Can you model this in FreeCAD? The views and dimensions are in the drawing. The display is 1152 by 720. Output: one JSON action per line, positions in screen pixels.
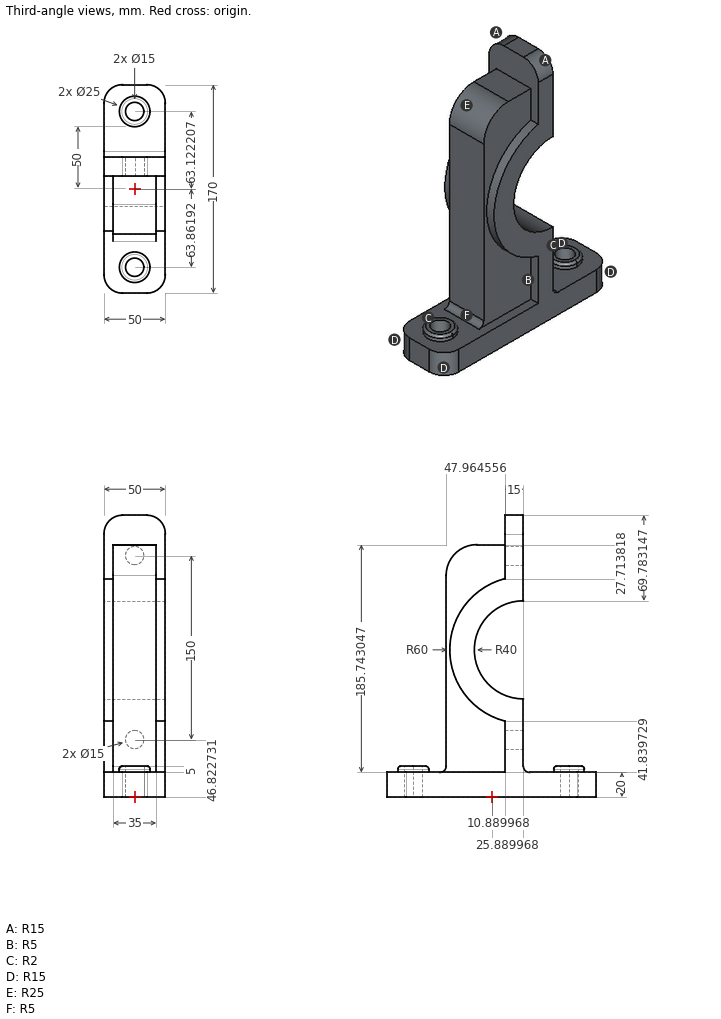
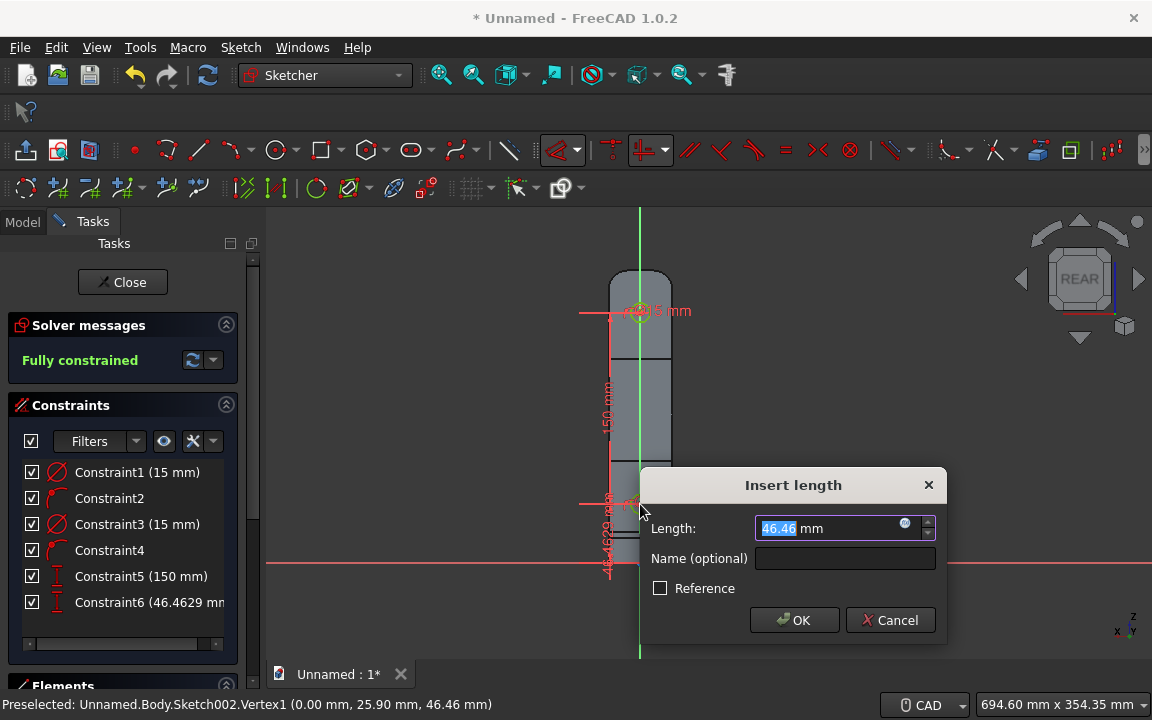
{"action": "type", "text": "46.822731"}
{"action": "key", "text": "Return"}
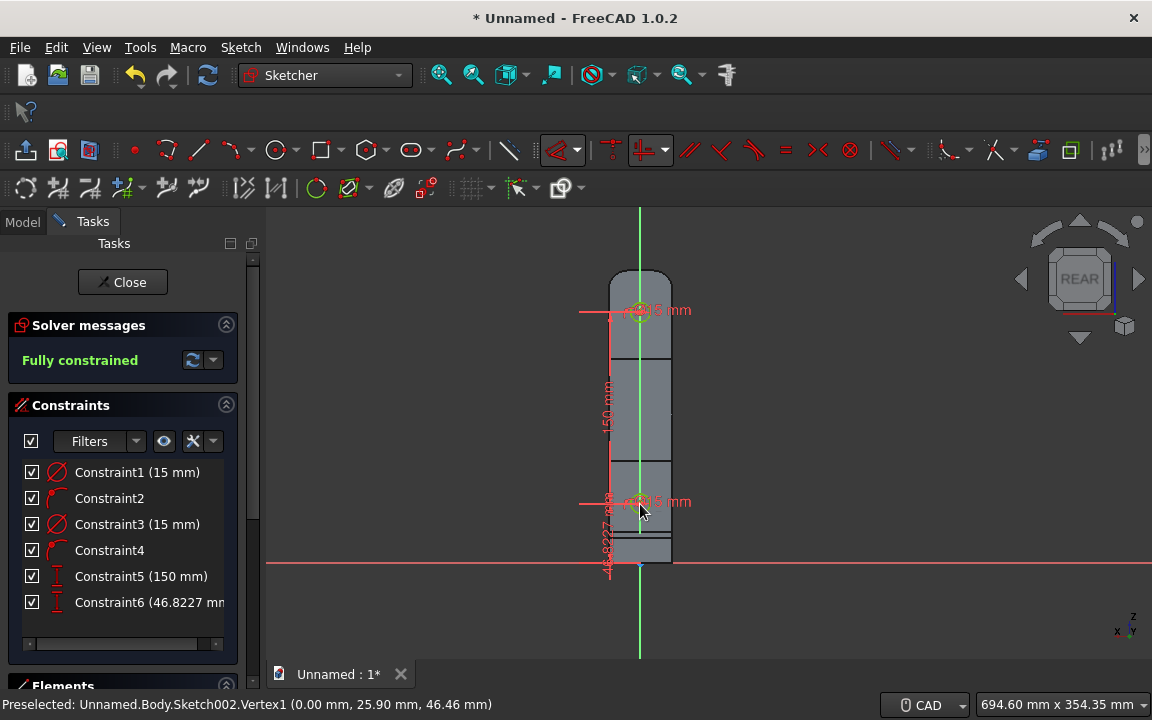
{"action": "left_click", "coordinate": [123, 282]}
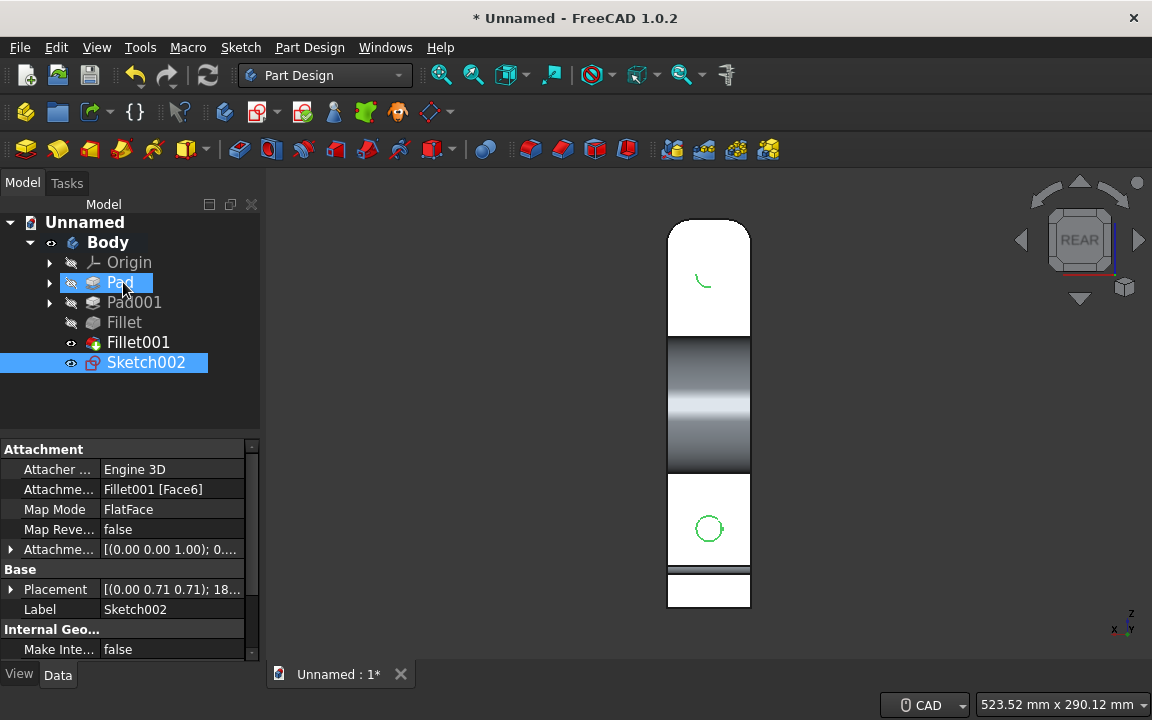
{"action": "left_click", "coordinate": [240, 150]}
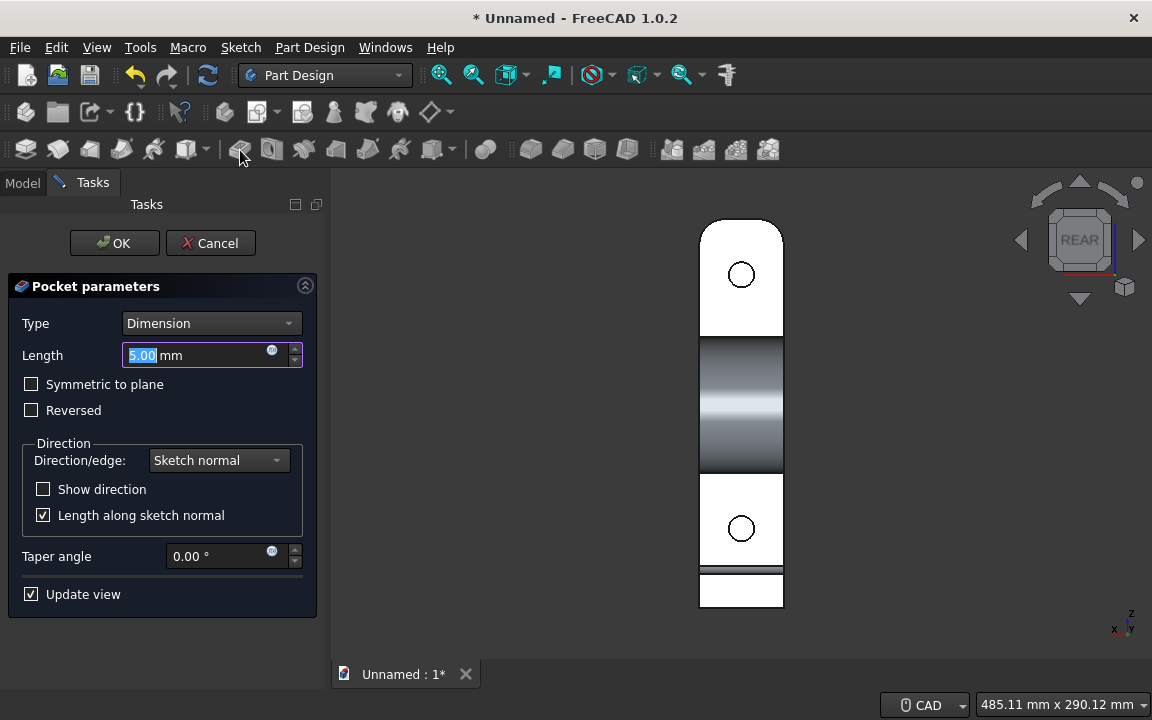
{"action": "type", "text": "50"}
{"action": "key", "text": "Tab"}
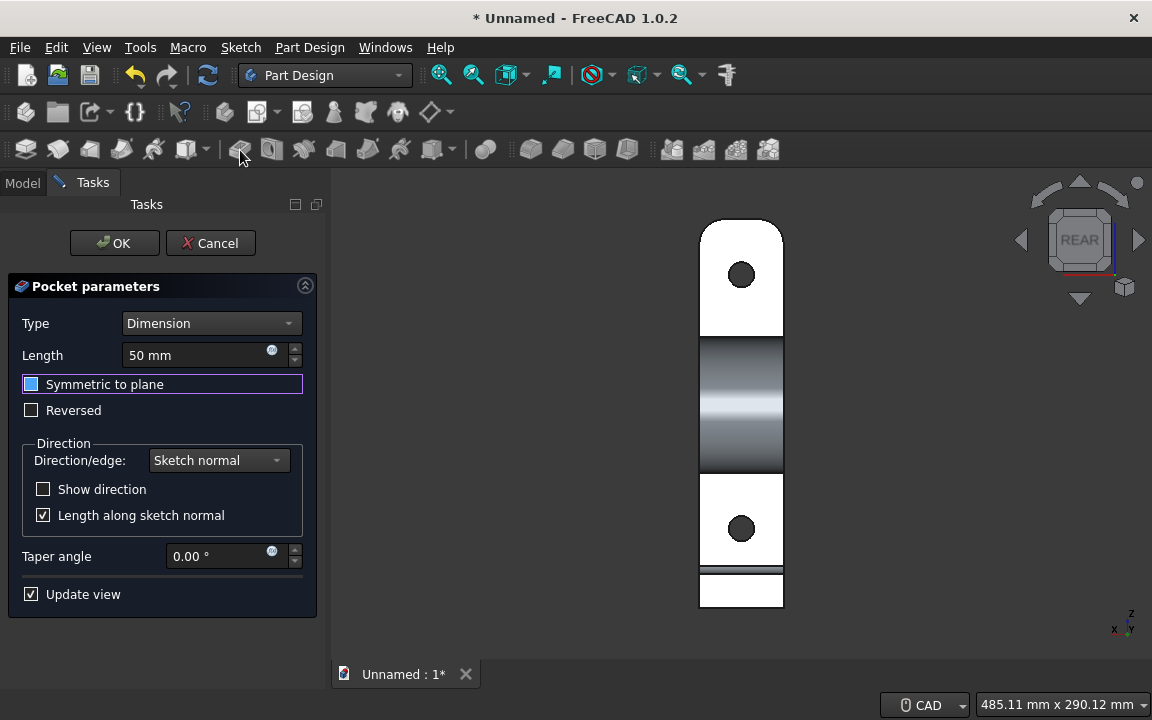
{"action": "left_click", "coordinate": [30, 384]}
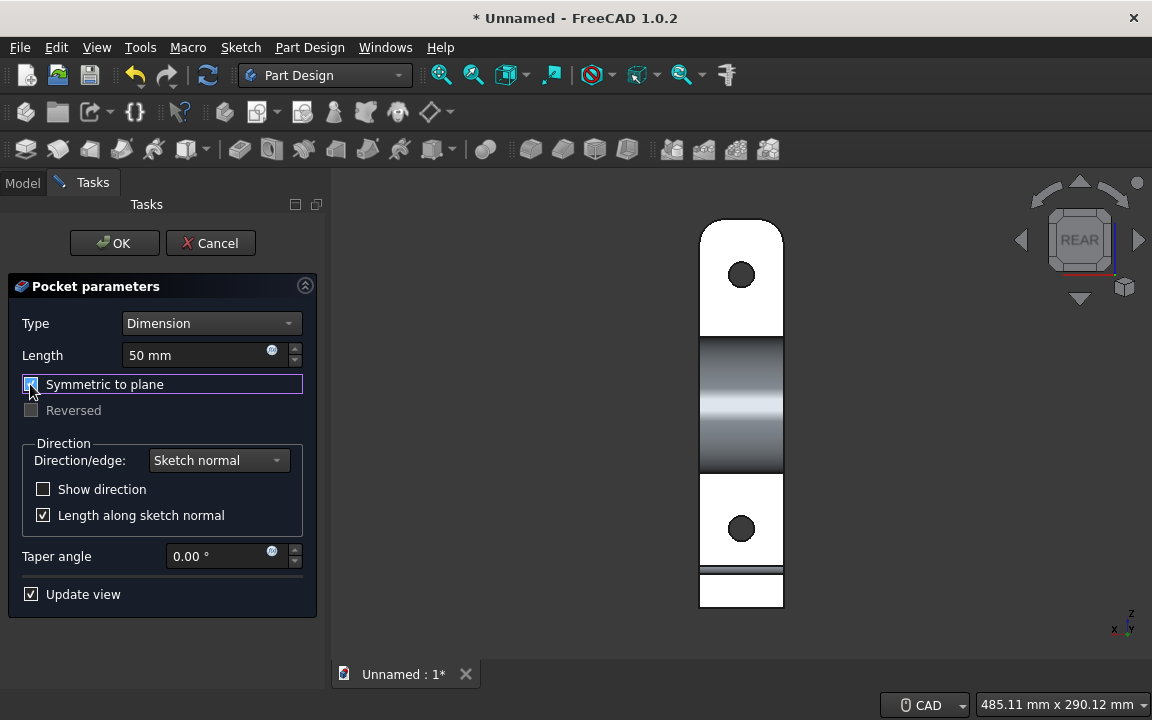
{"action": "left_click", "coordinate": [115, 243]}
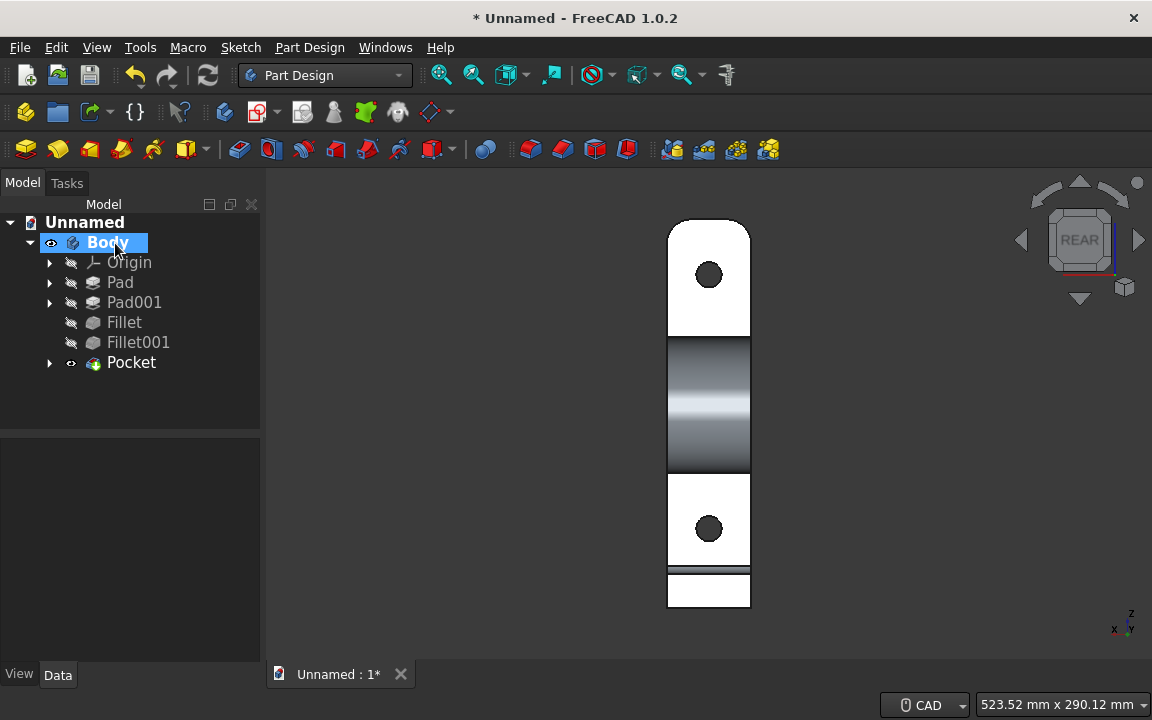
{"action": "key", "text": "0"}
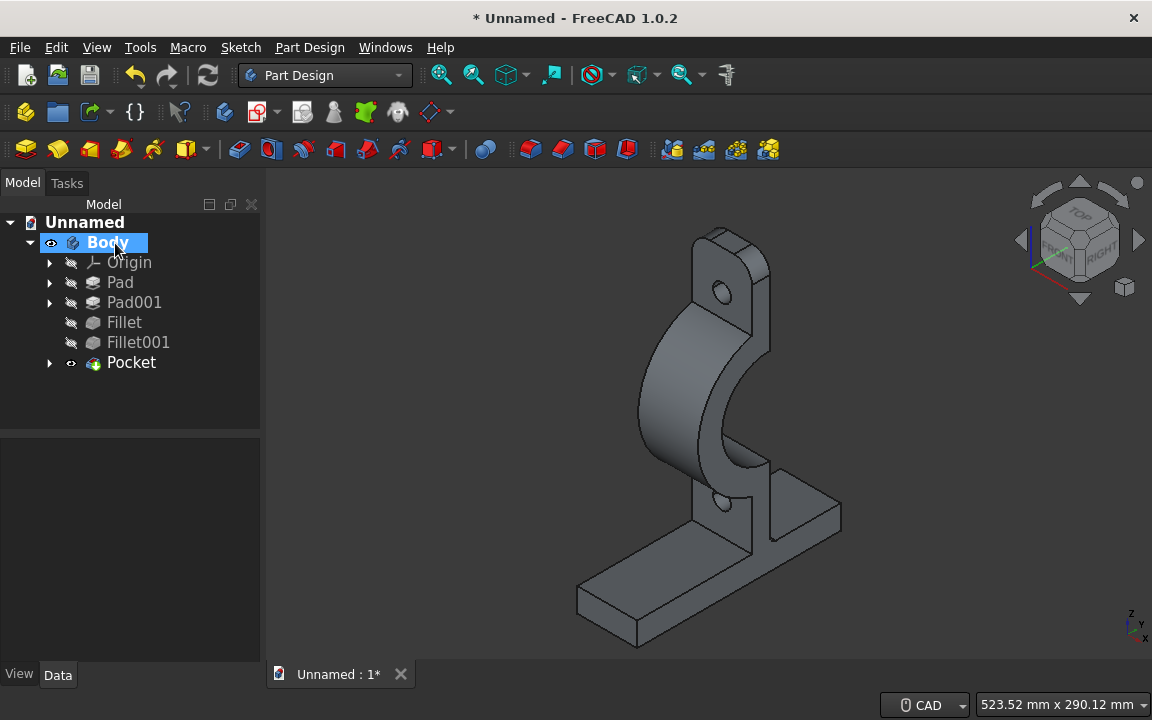
{"action": "left_click", "coordinate": [665, 569]}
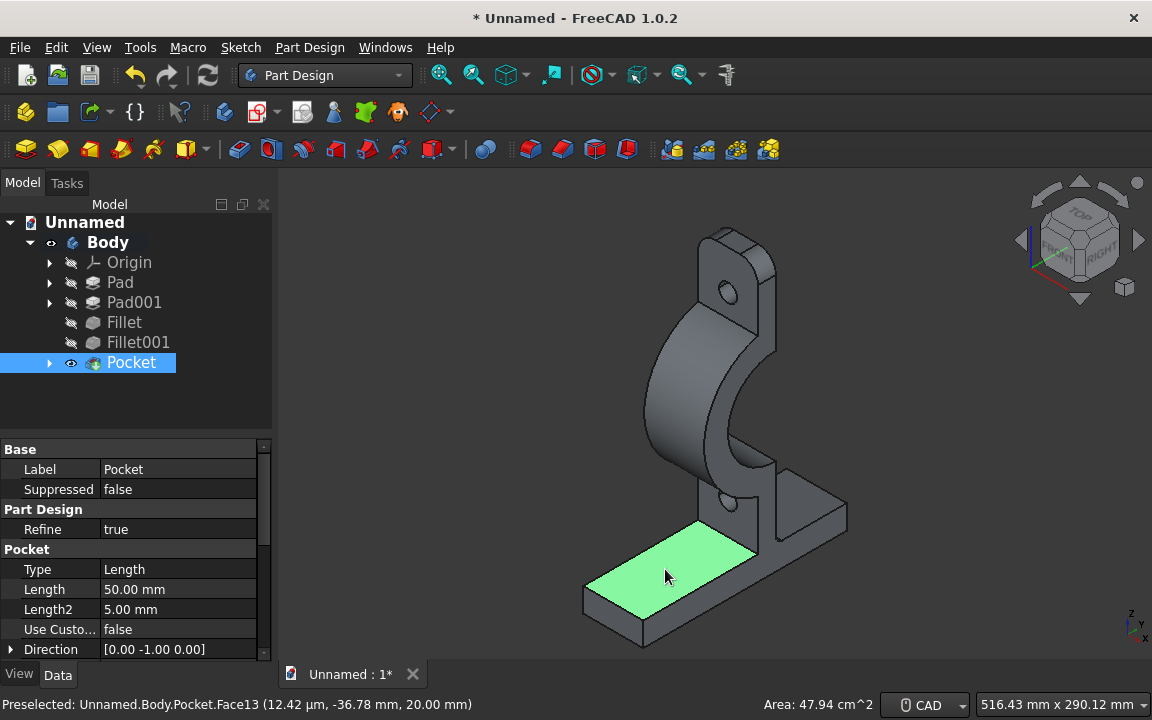
{"action": "left_click", "coordinate": [258, 112]}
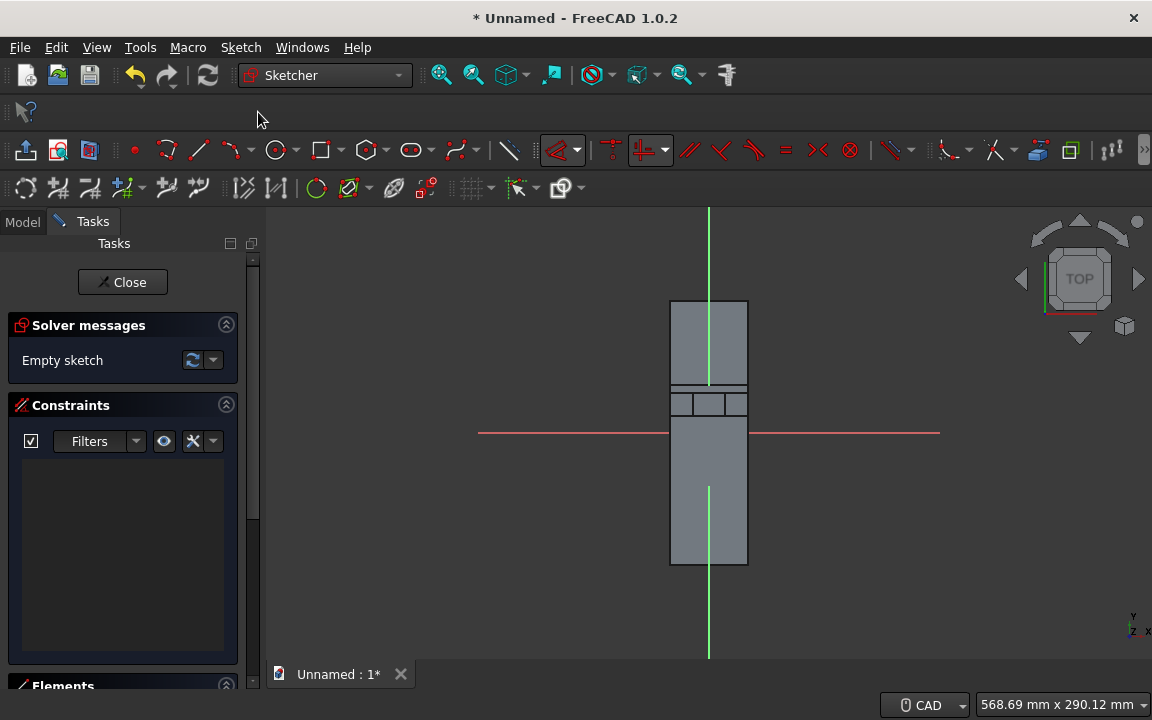
{"action": "key", "text": "q s"}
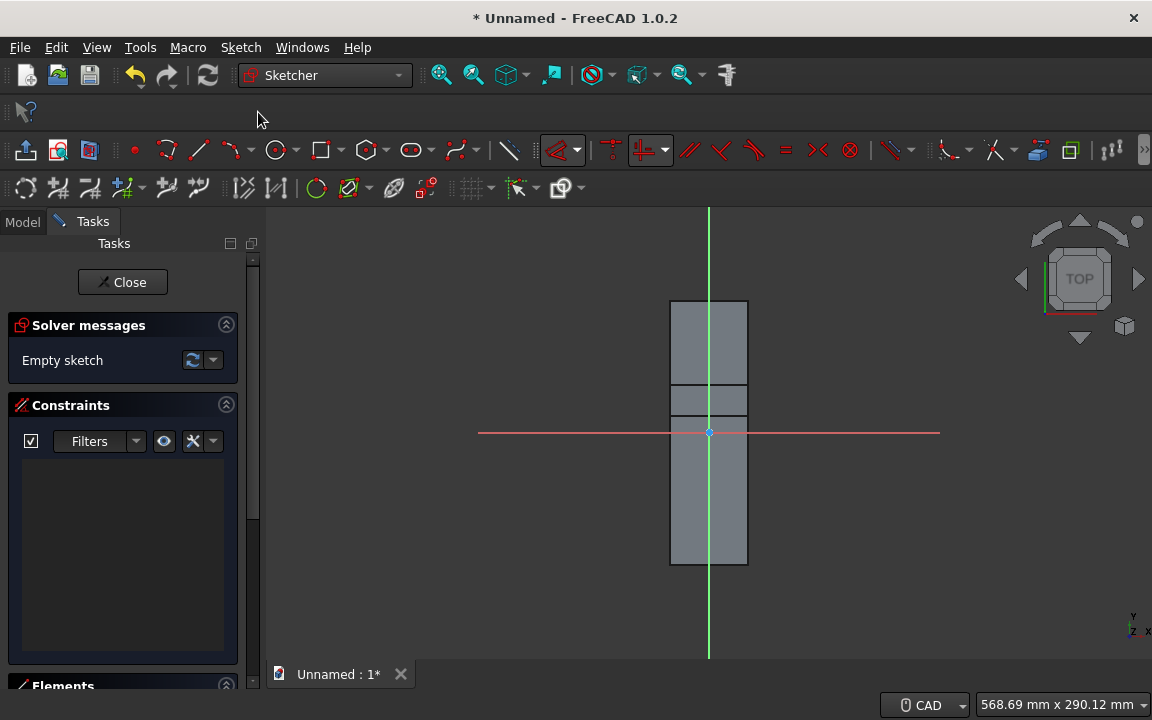
{"action": "left_click", "coordinate": [276, 150]}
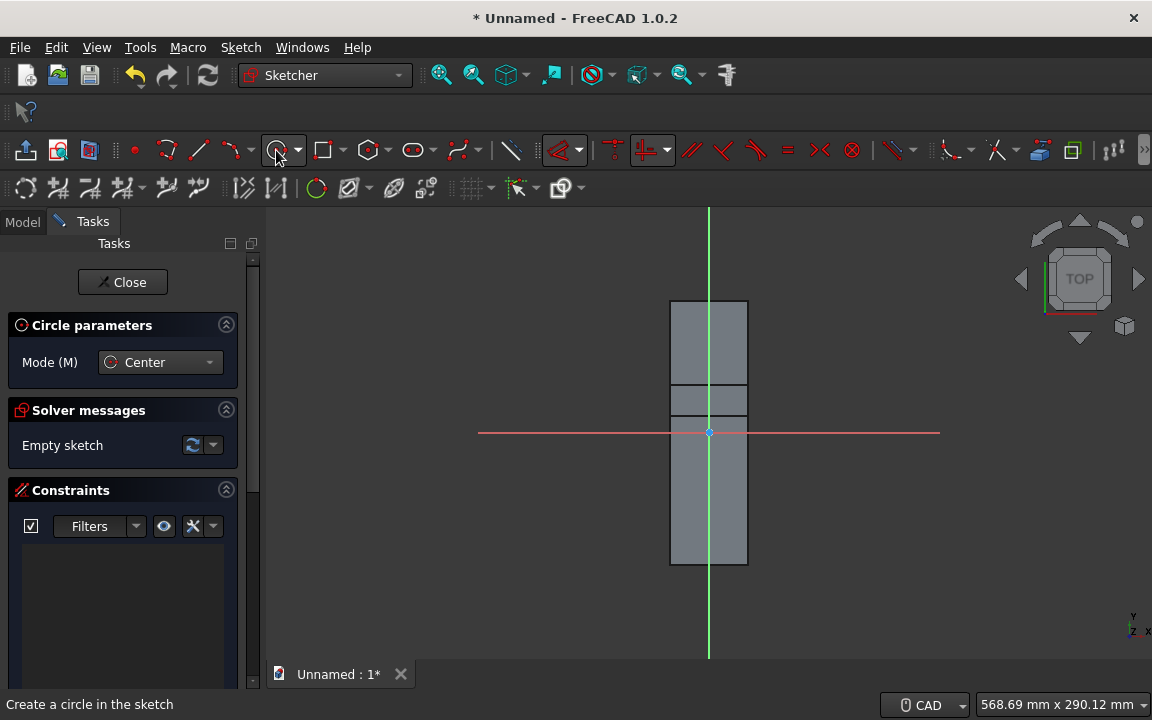
{"action": "scroll", "coordinate": [709, 335], "scroll_direction": "up", "scroll_amount": 4}